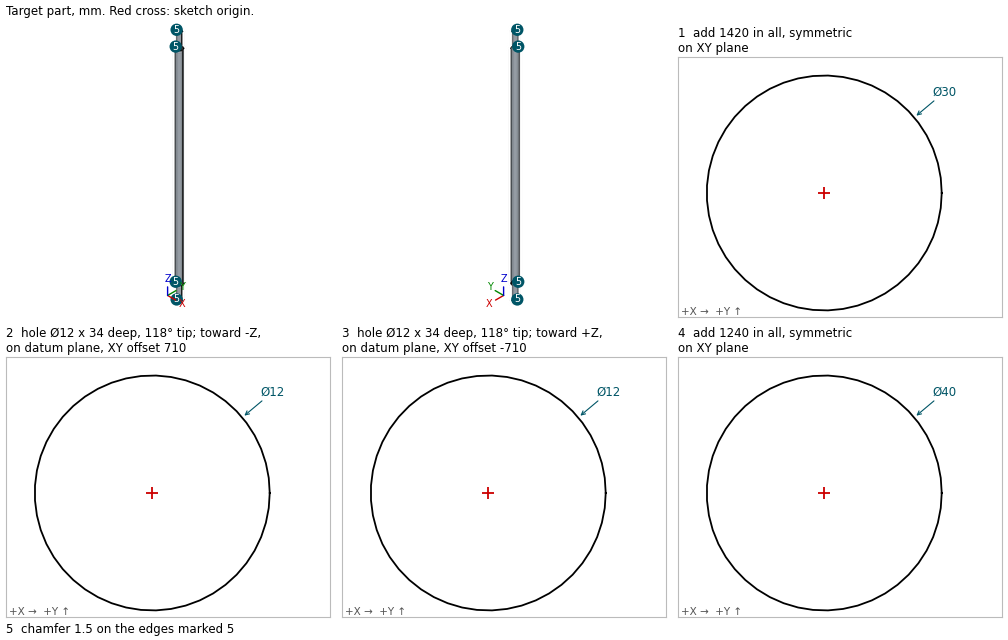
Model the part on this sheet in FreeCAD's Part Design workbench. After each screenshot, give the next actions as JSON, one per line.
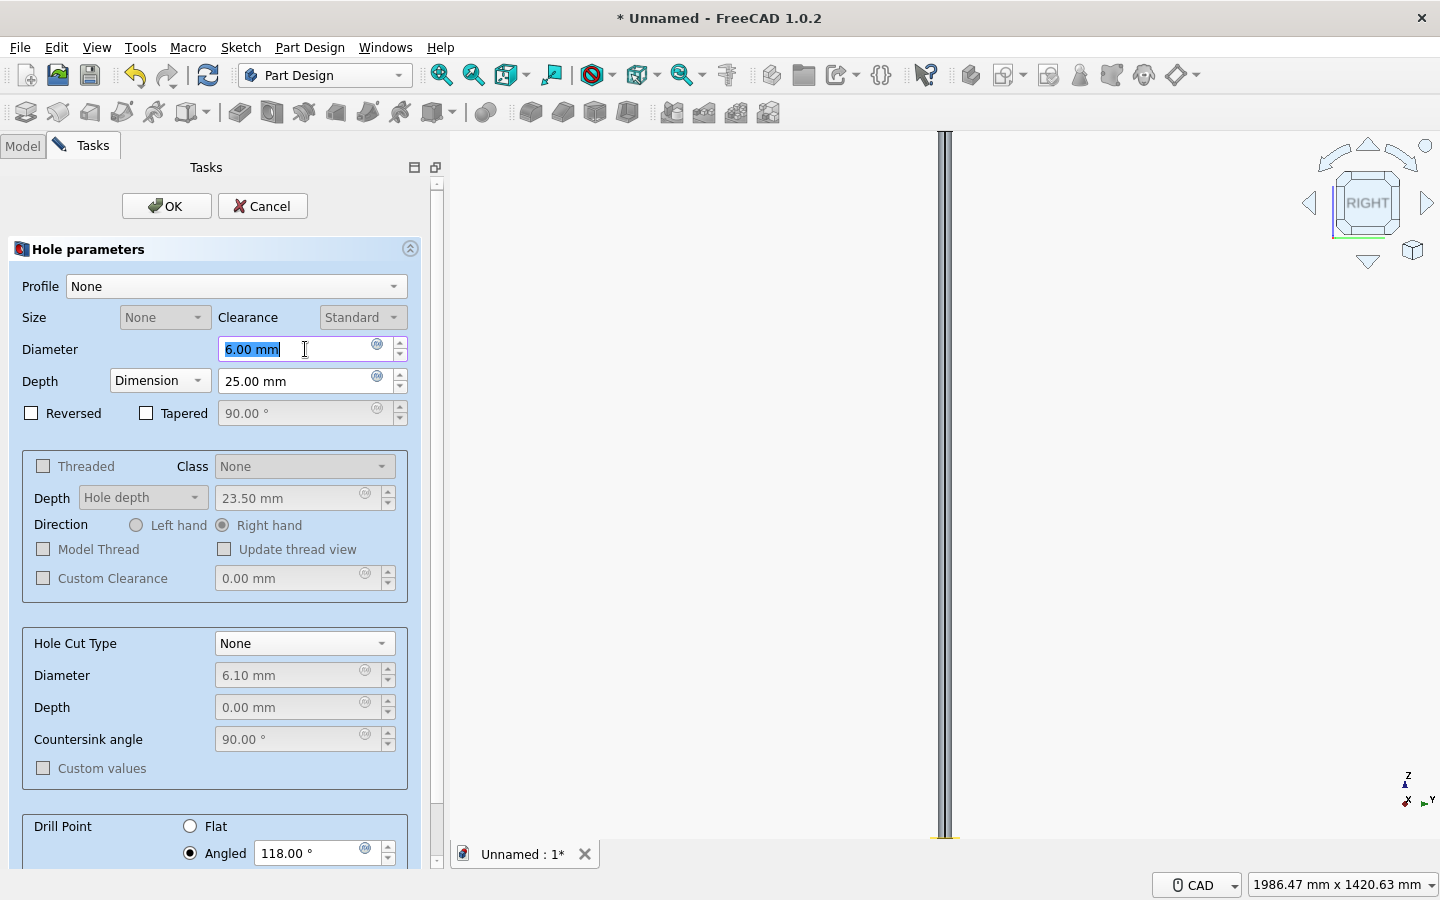
{"action": "type", "text": "12"}
{"action": "key", "text": "Tab"}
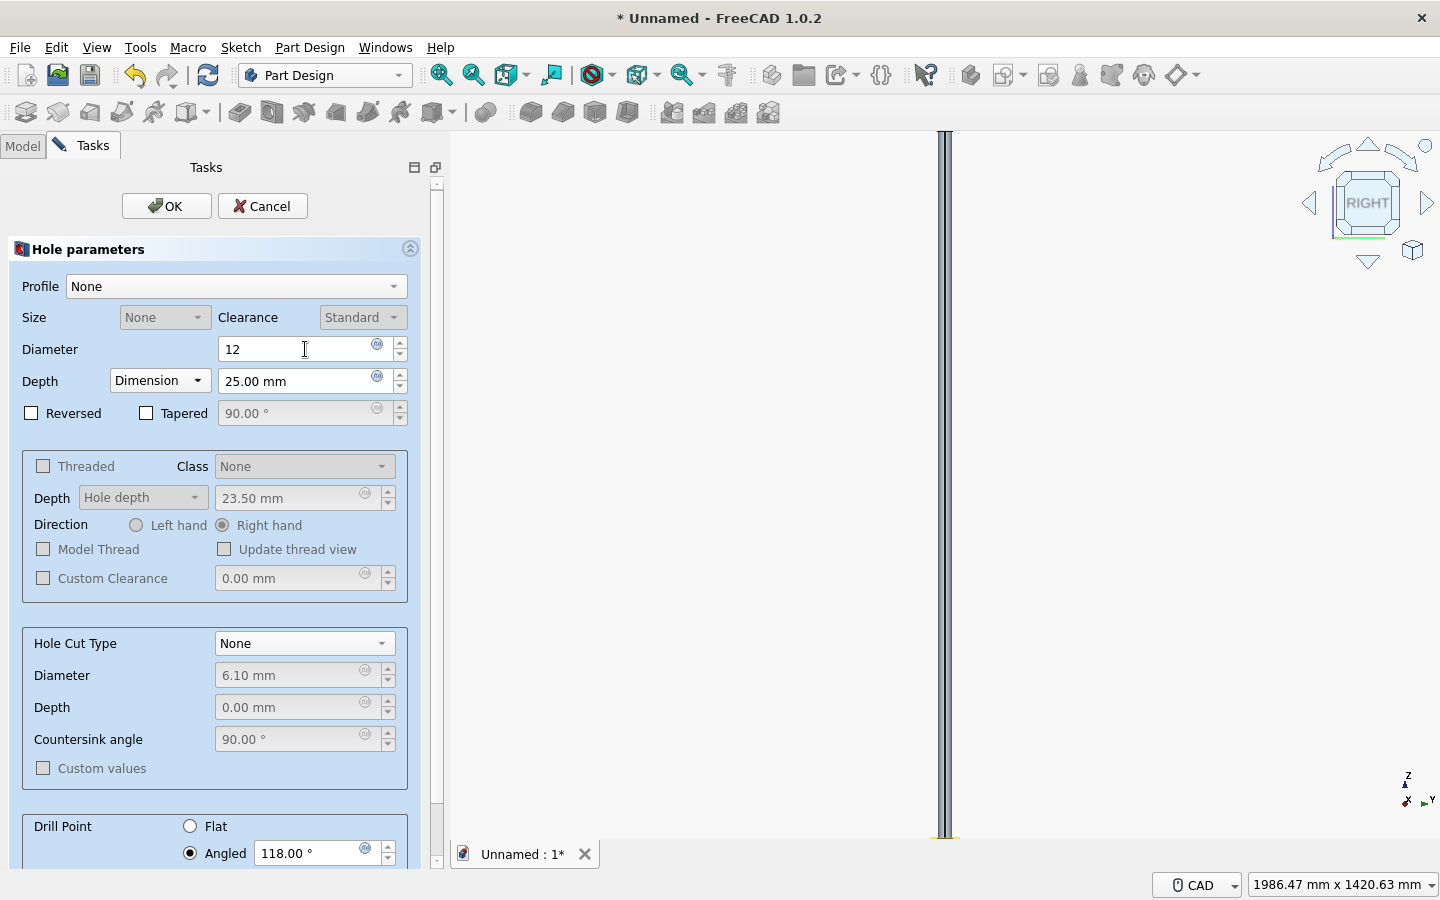
{"action": "triple_click", "coordinate": [305, 381]}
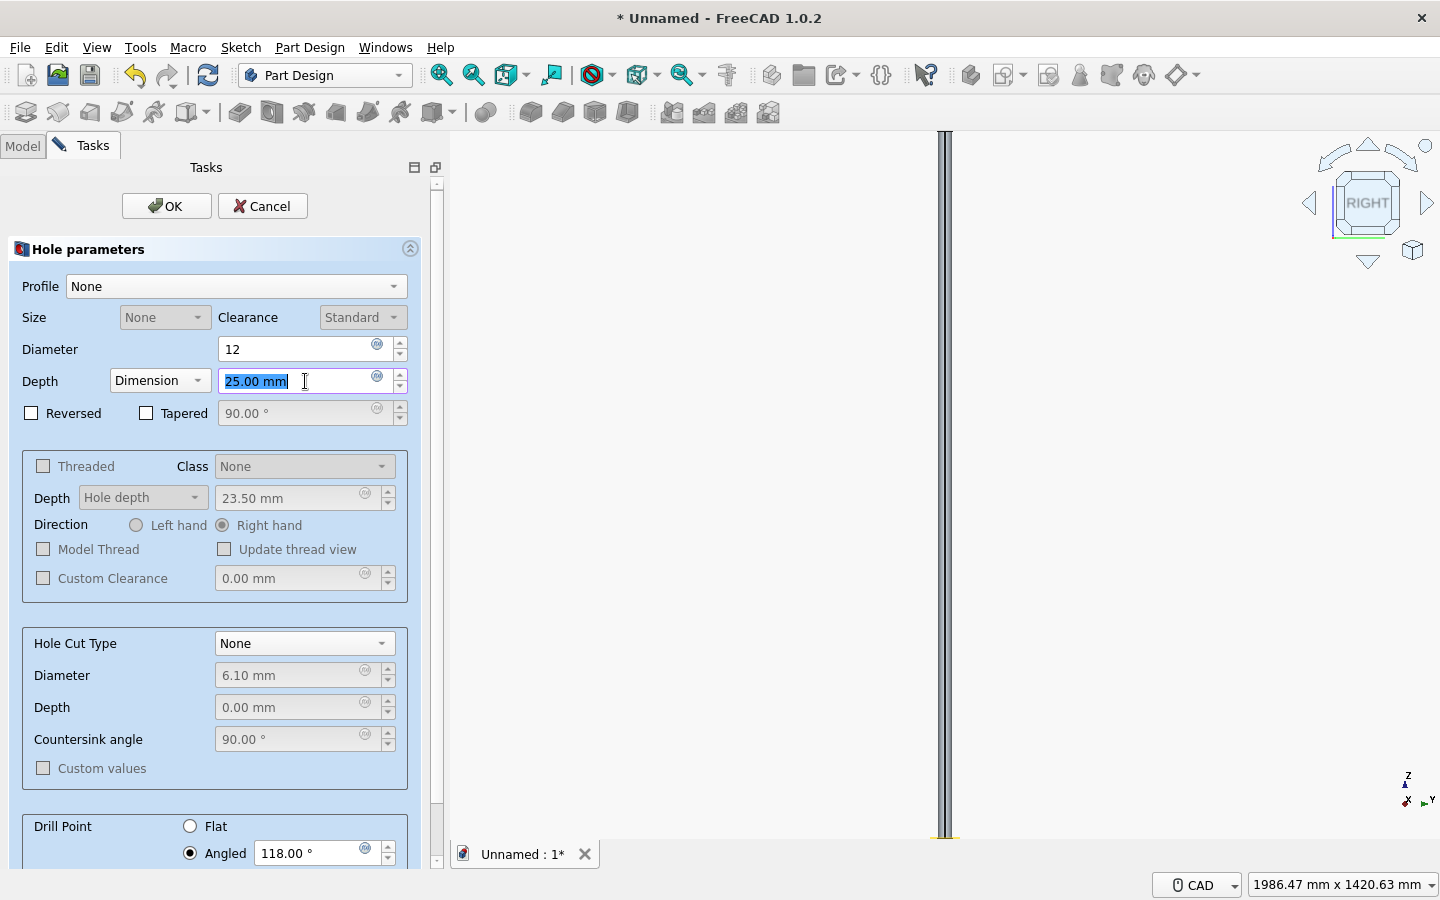
{"action": "type", "text": "34"}
{"action": "key", "text": "Tab"}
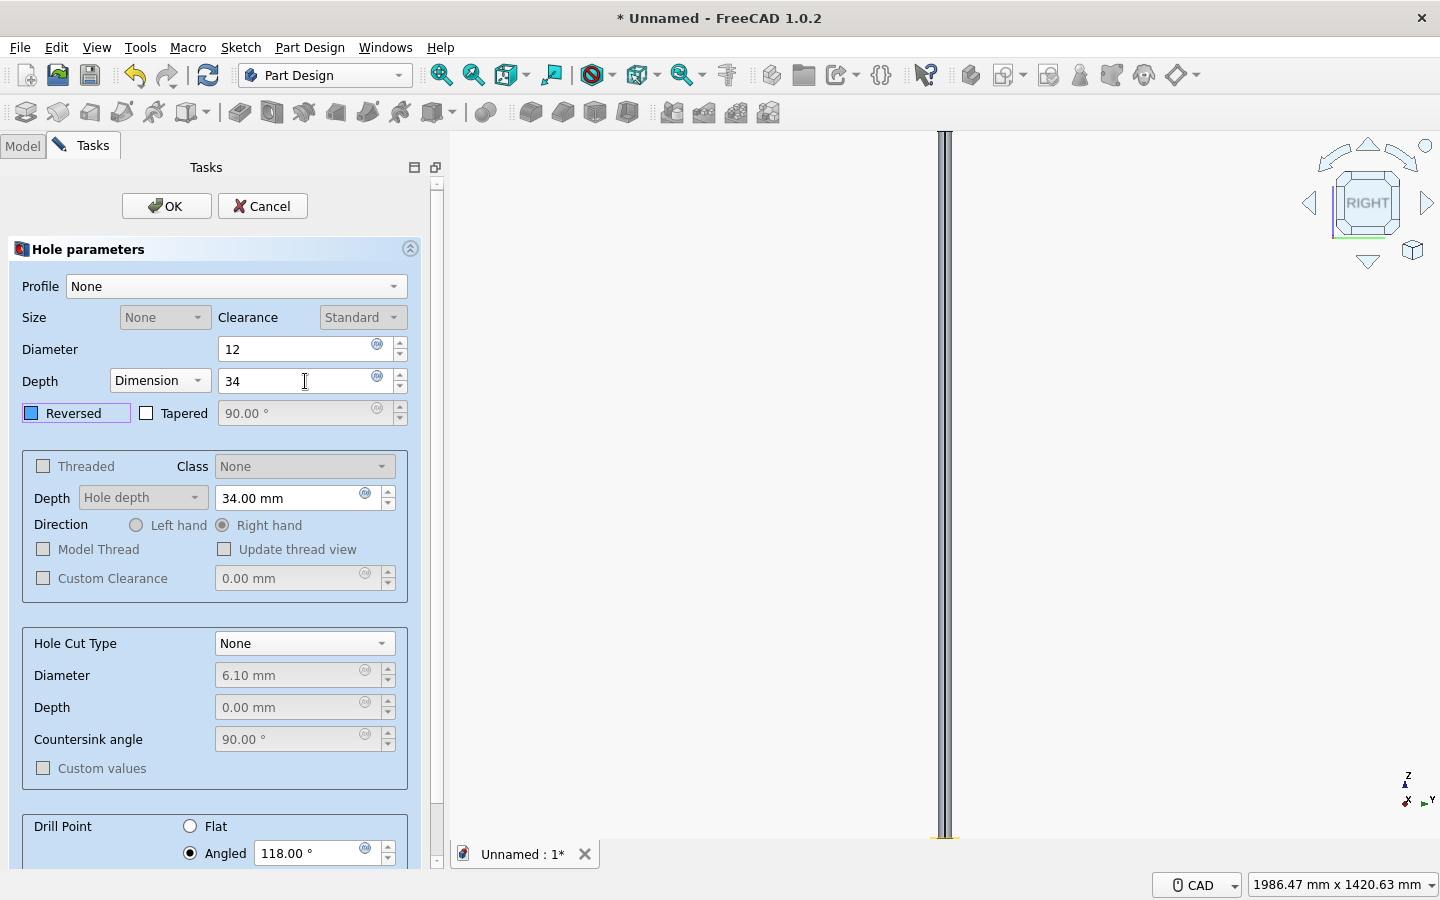
{"action": "left_click", "coordinate": [30, 413]}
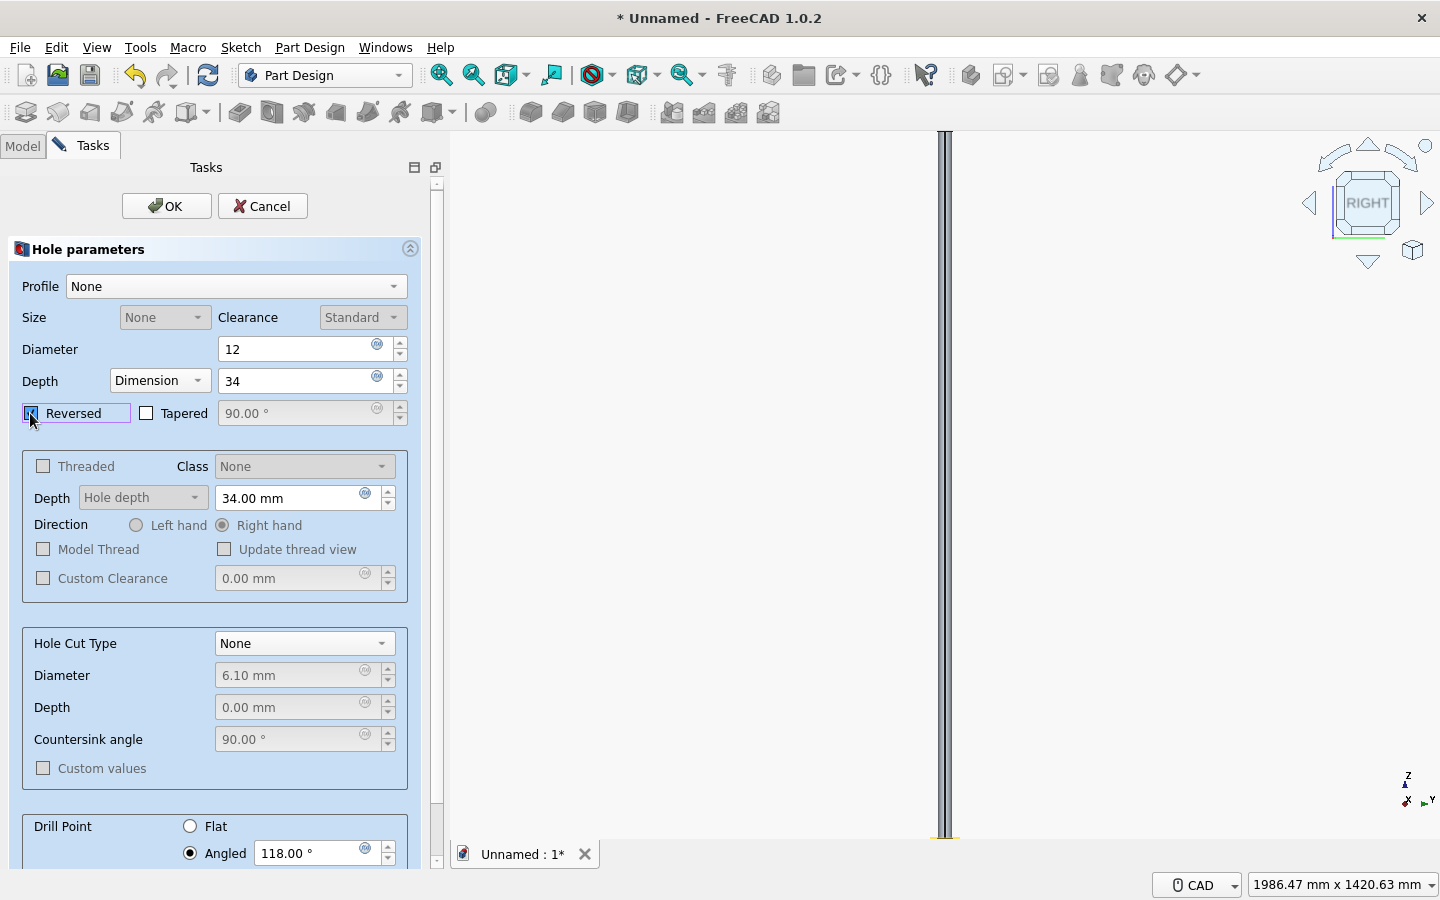
{"action": "left_click", "coordinate": [167, 206]}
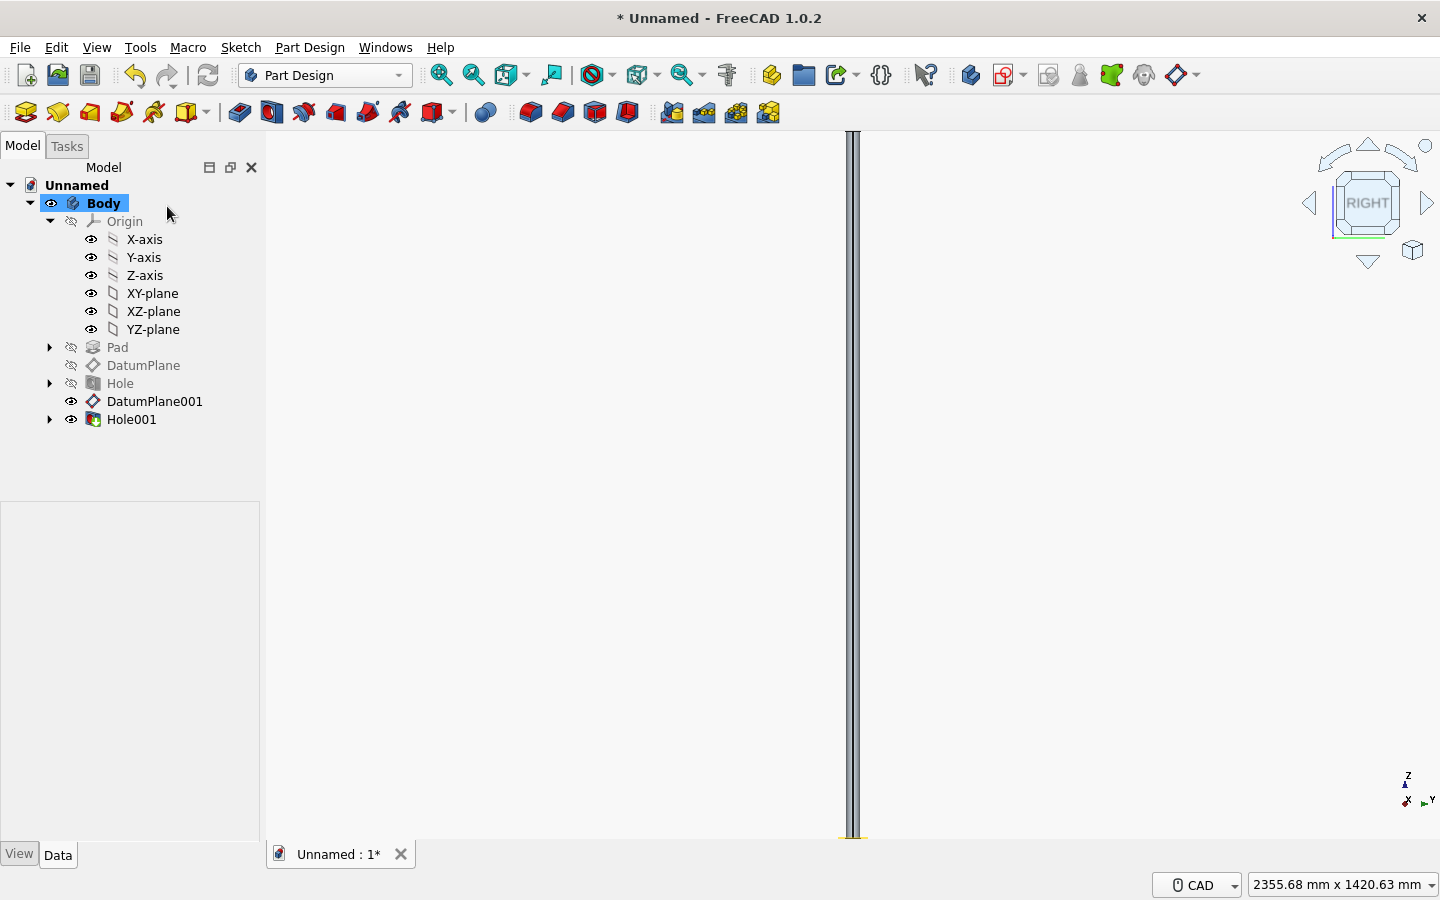
{"action": "left_click", "coordinate": [116, 401]}
{"action": "key", "text": "space"}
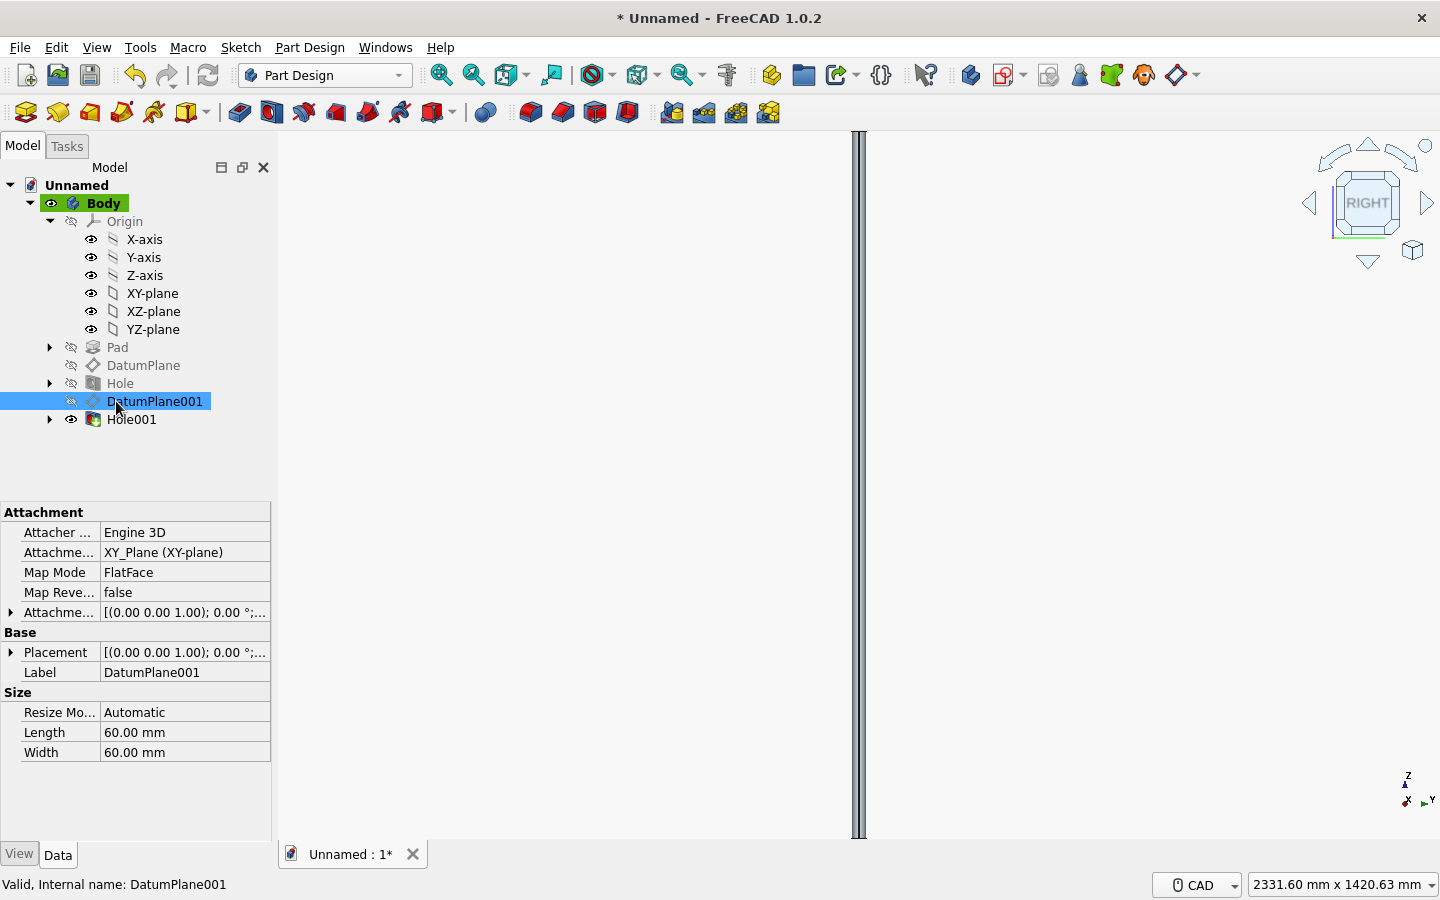
{"action": "left_click", "coordinate": [442, 76]}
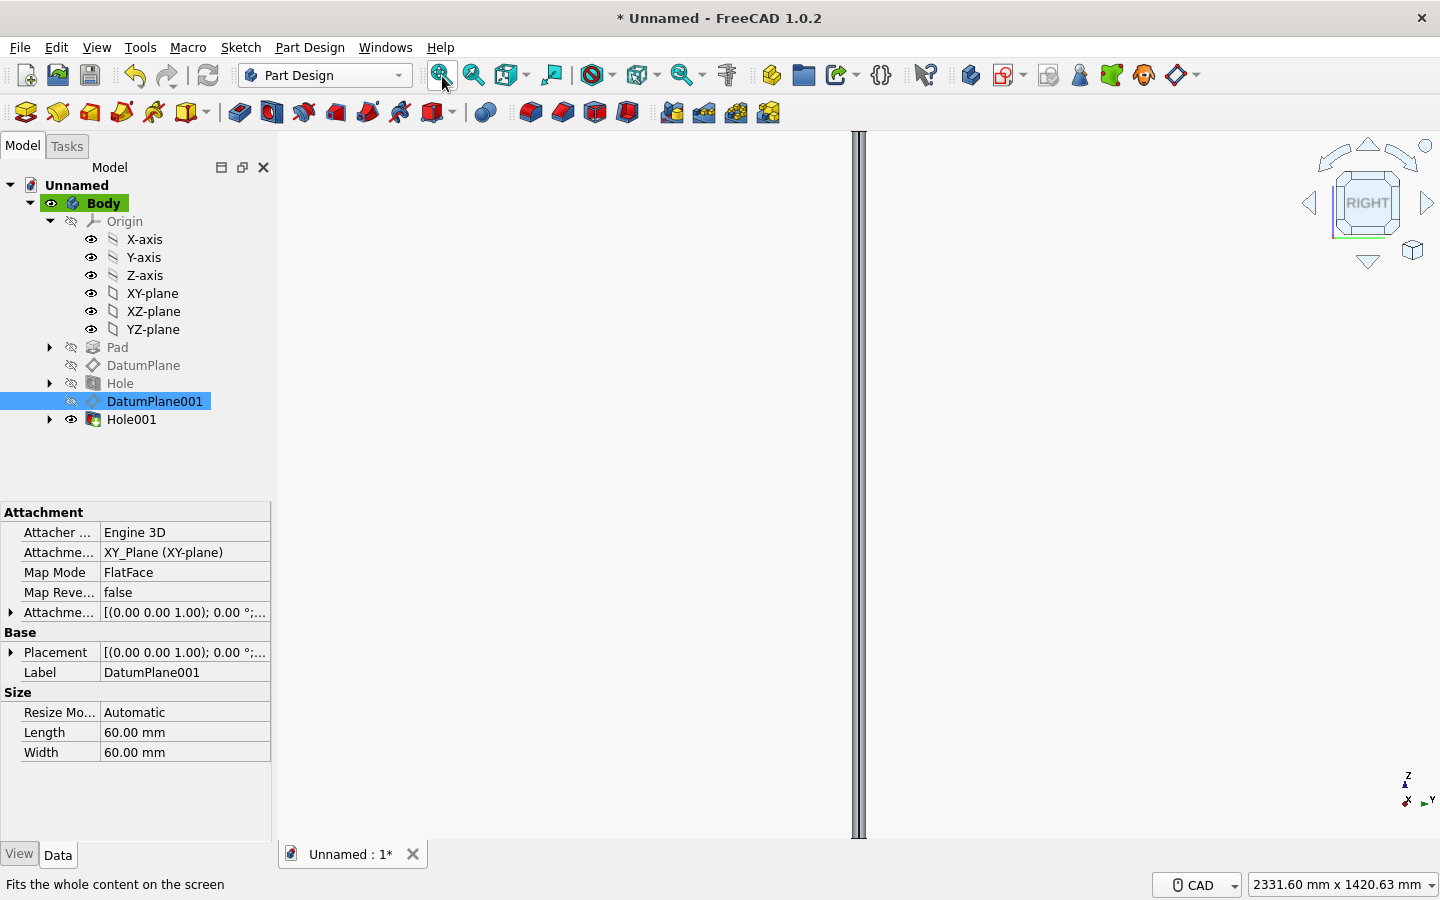
{"action": "left_click", "coordinate": [318, 799]}